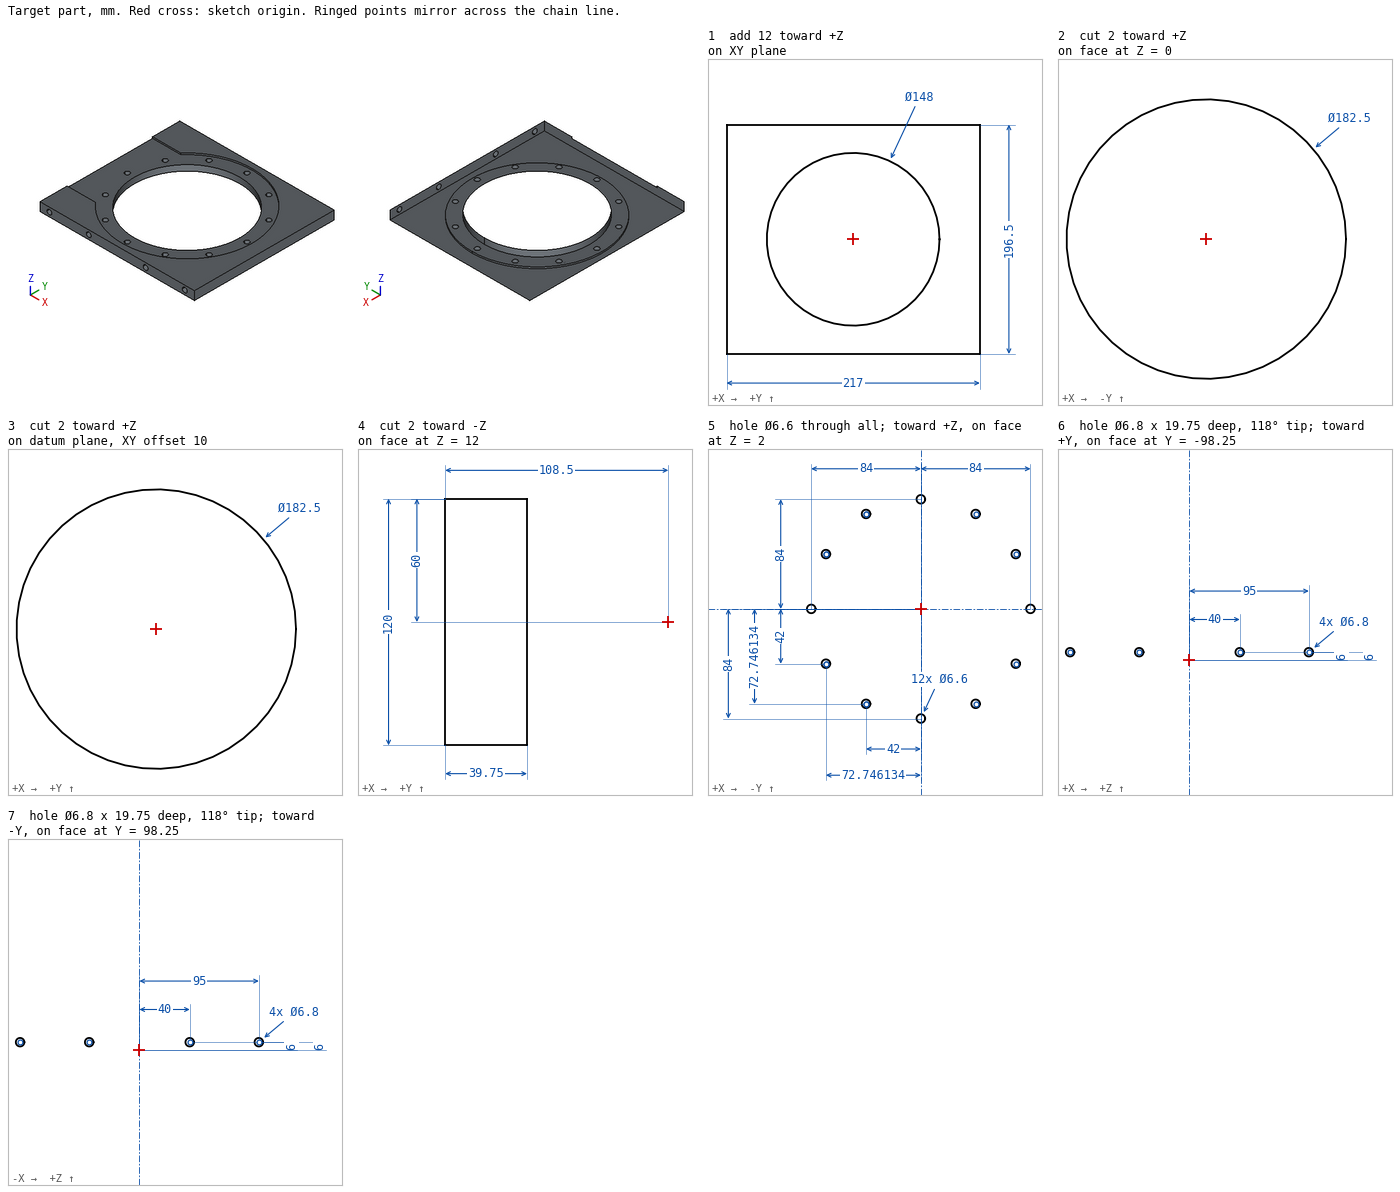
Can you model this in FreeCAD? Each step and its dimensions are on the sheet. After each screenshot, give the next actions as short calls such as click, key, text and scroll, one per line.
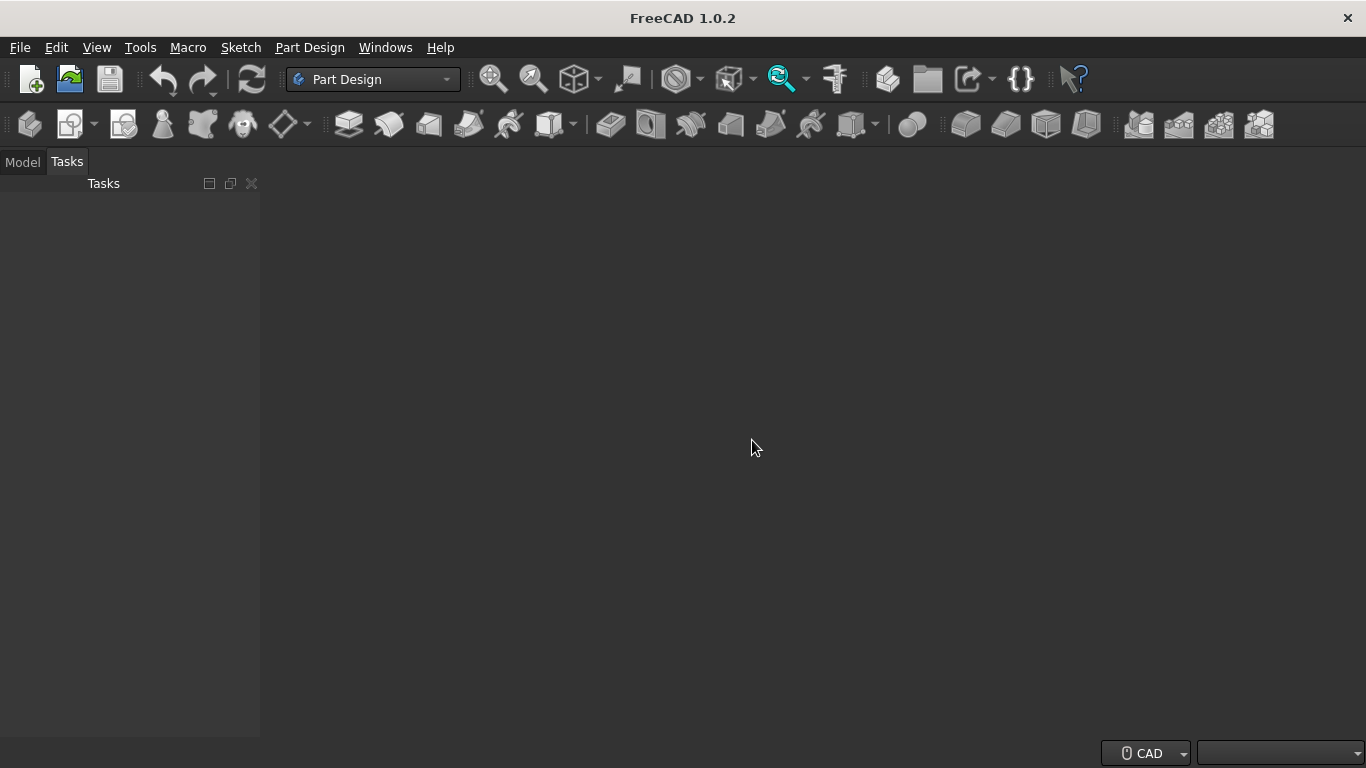
click(30, 80)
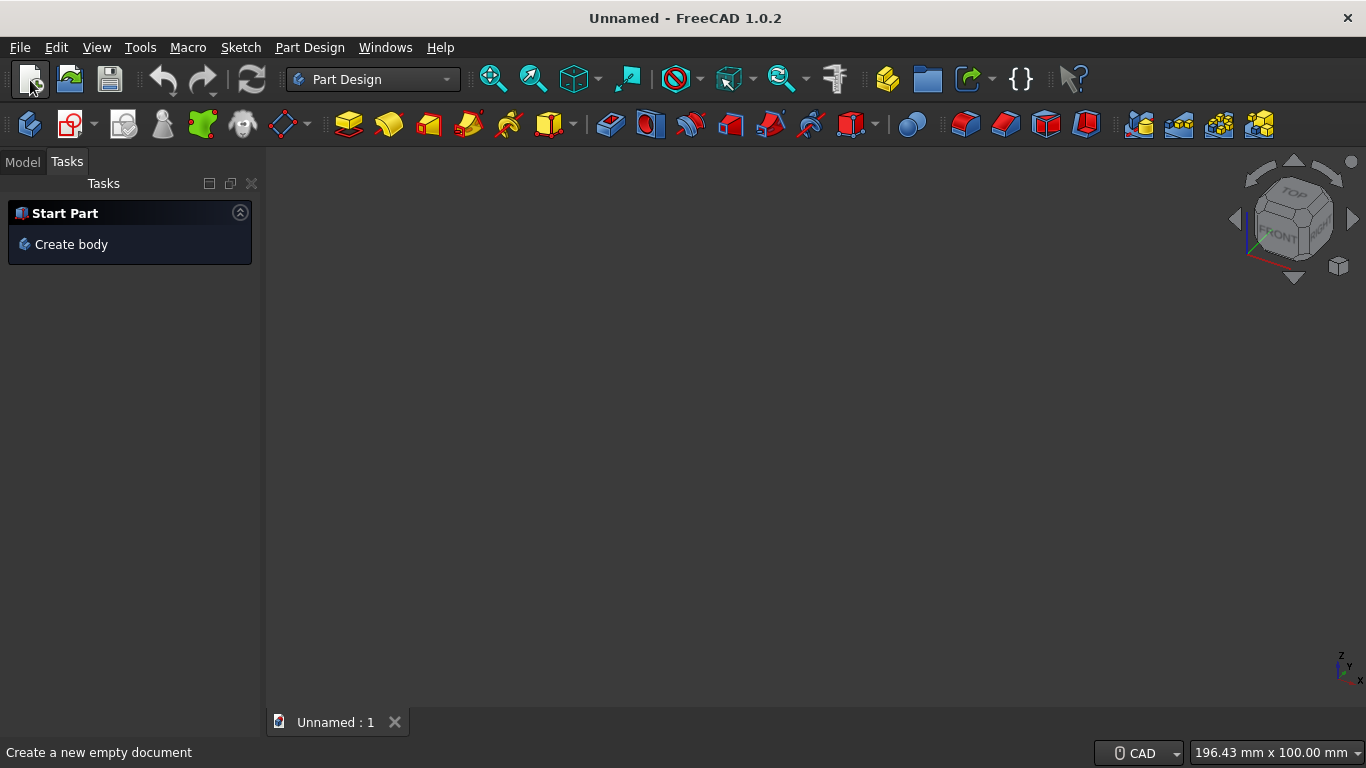
click(70, 124)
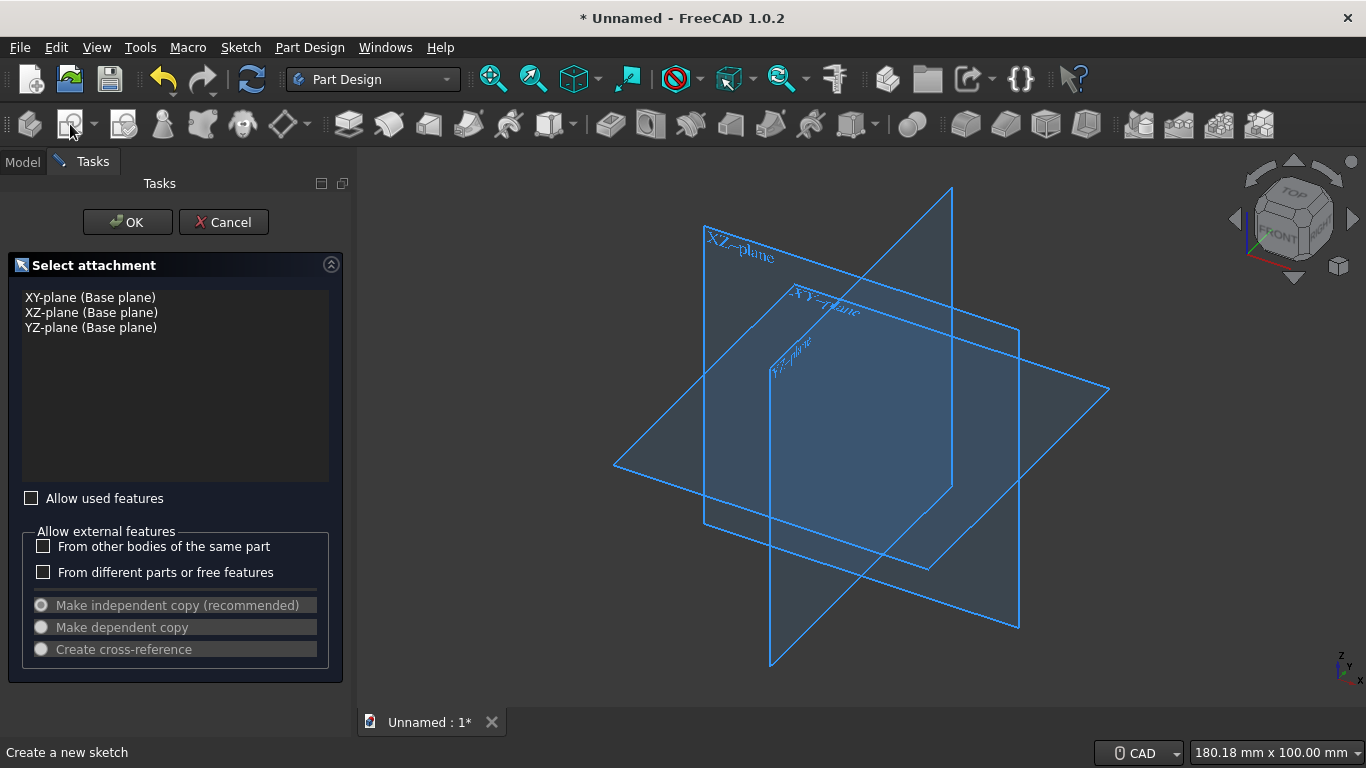
click(82, 298)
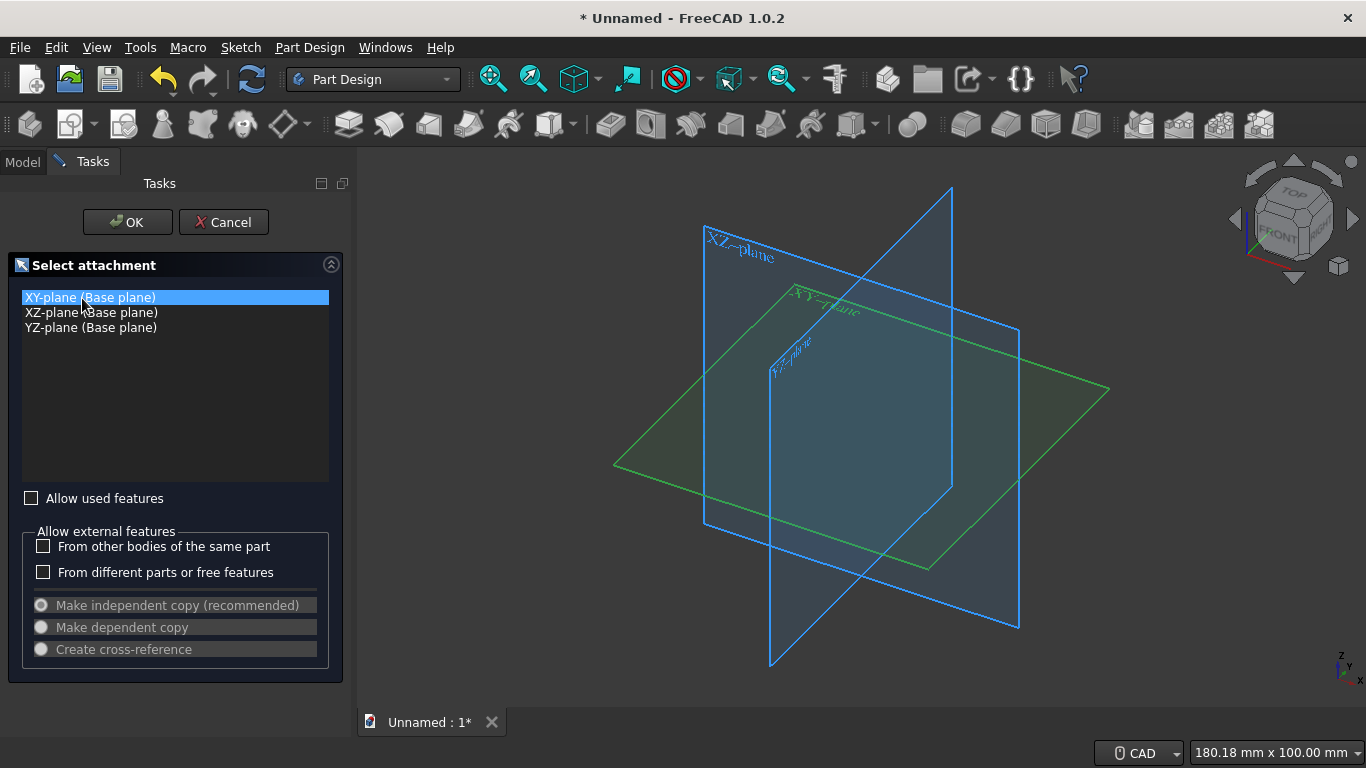
click(128, 222)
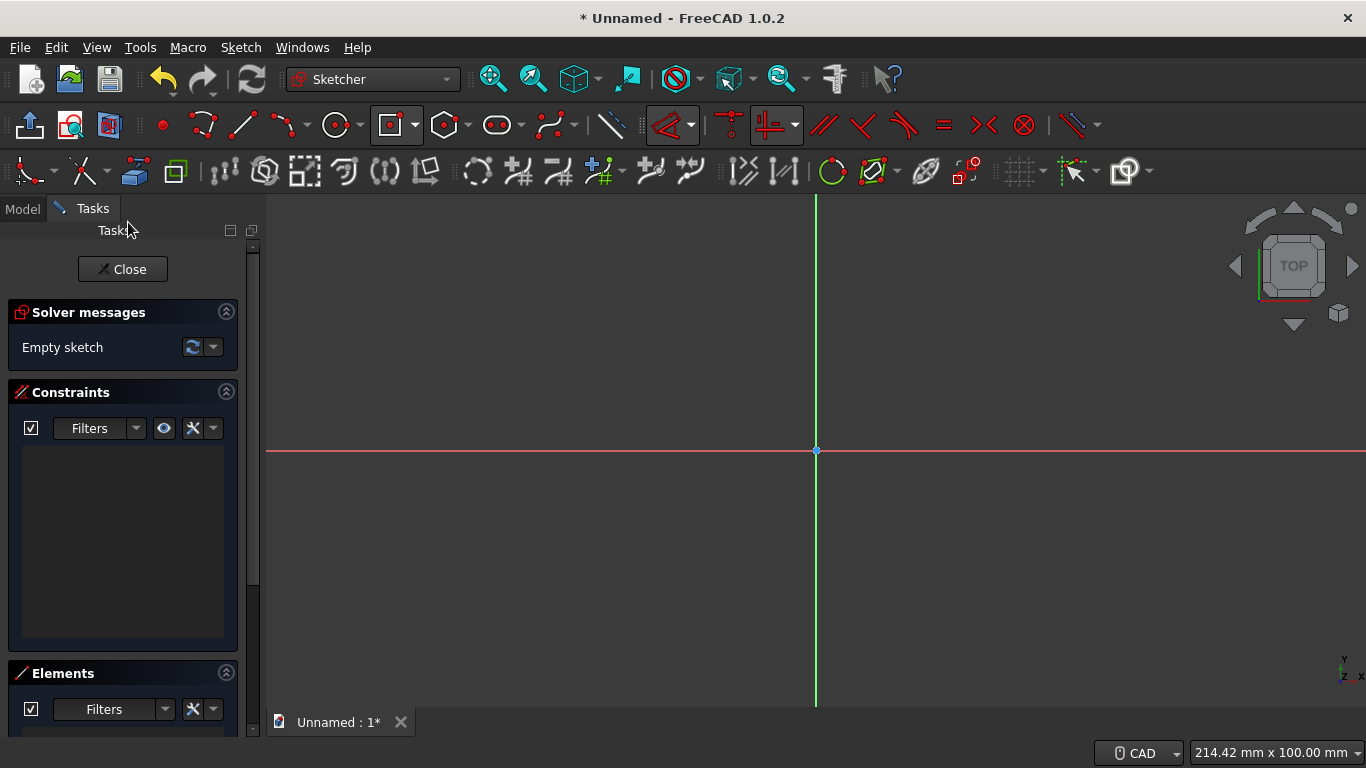
scroll(718, 450, down, 6)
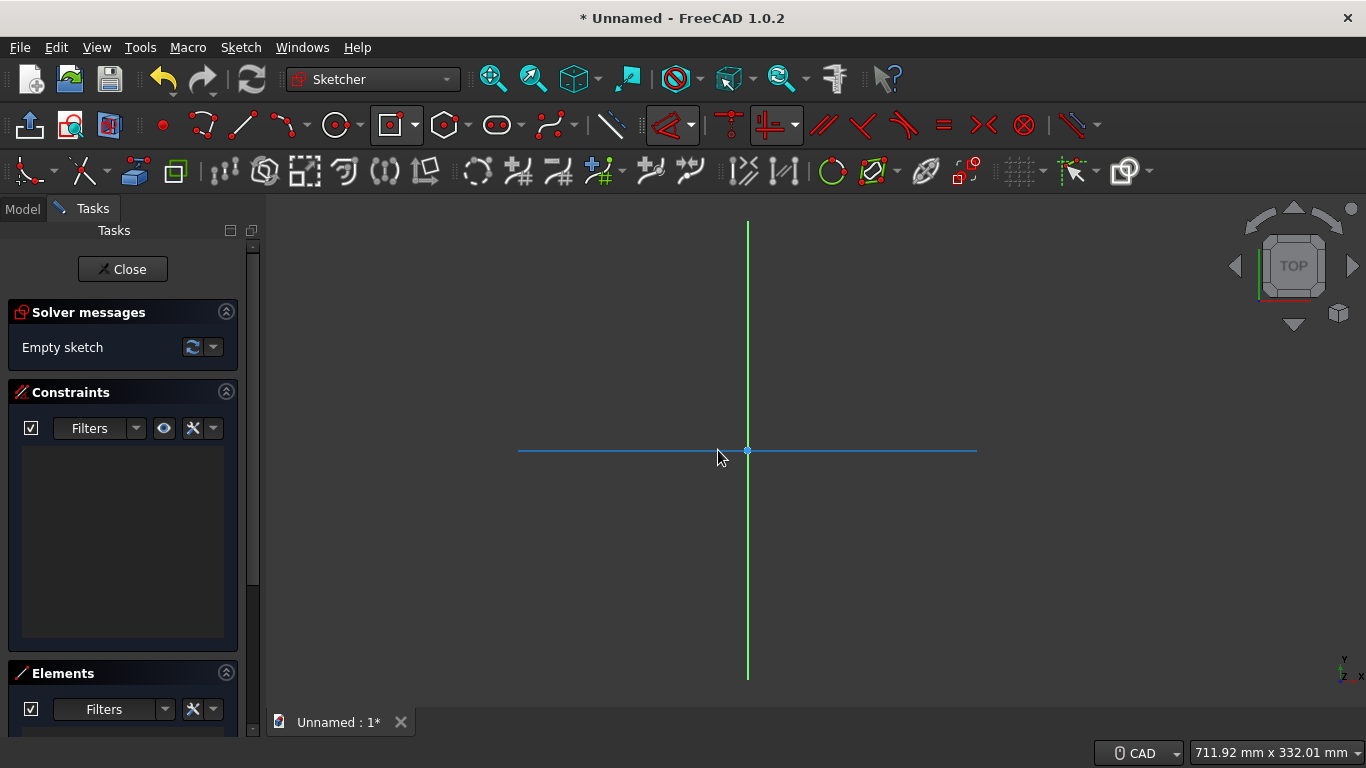
click(390, 126)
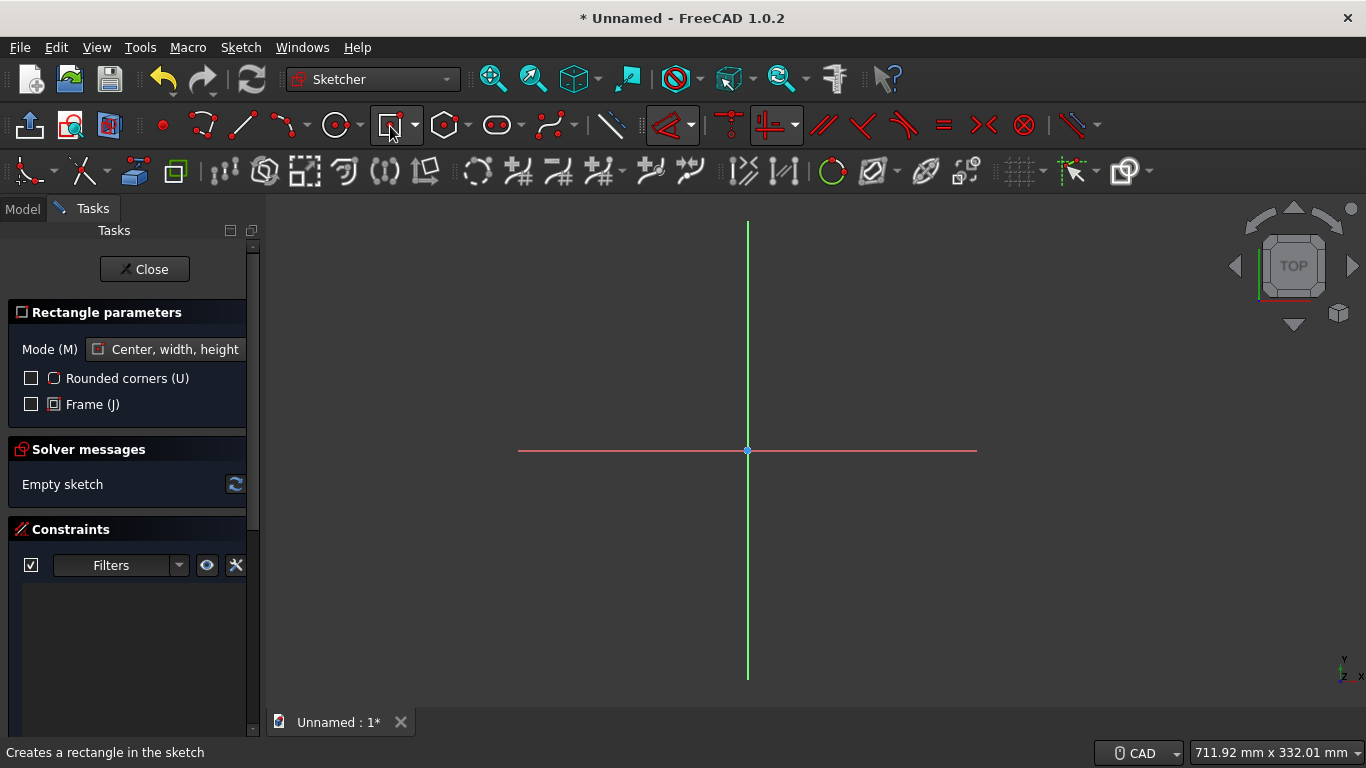
click(748, 450)
click(915, 299)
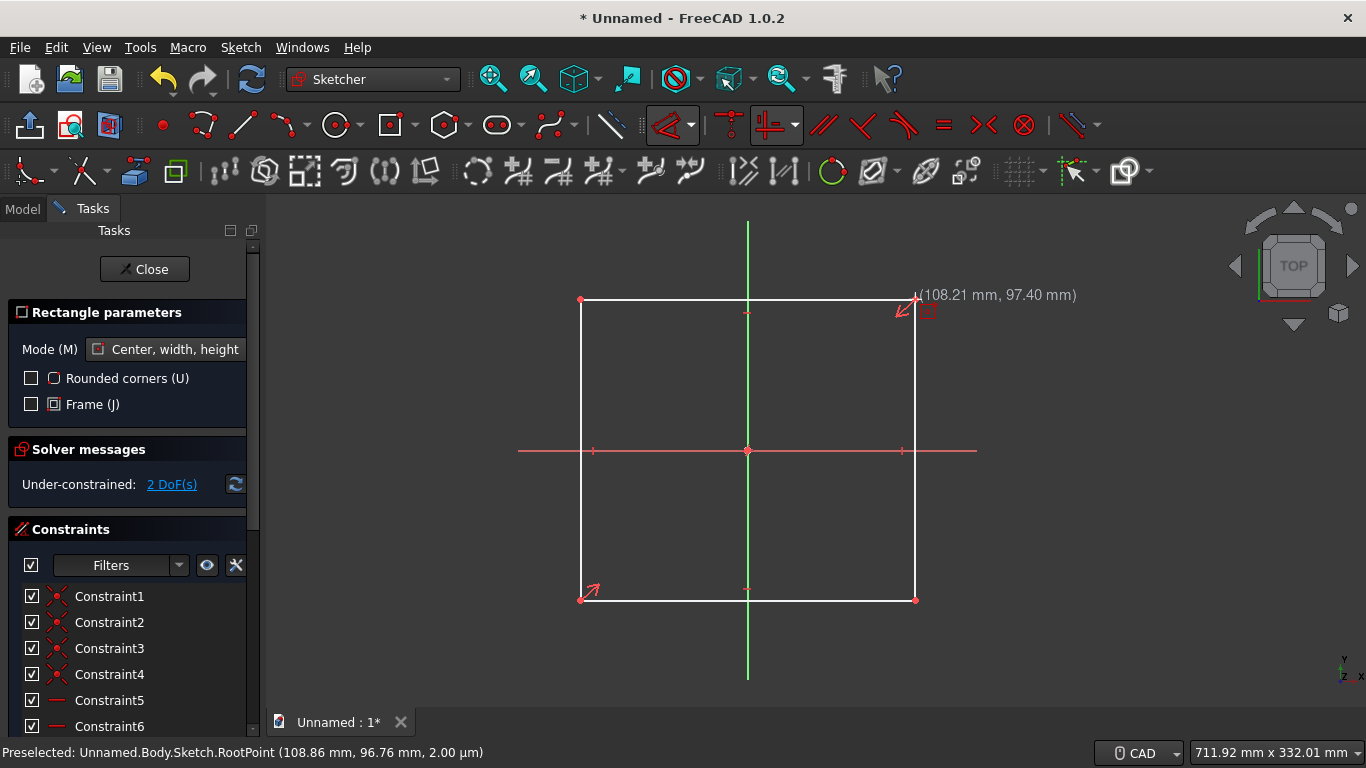
click(336, 126)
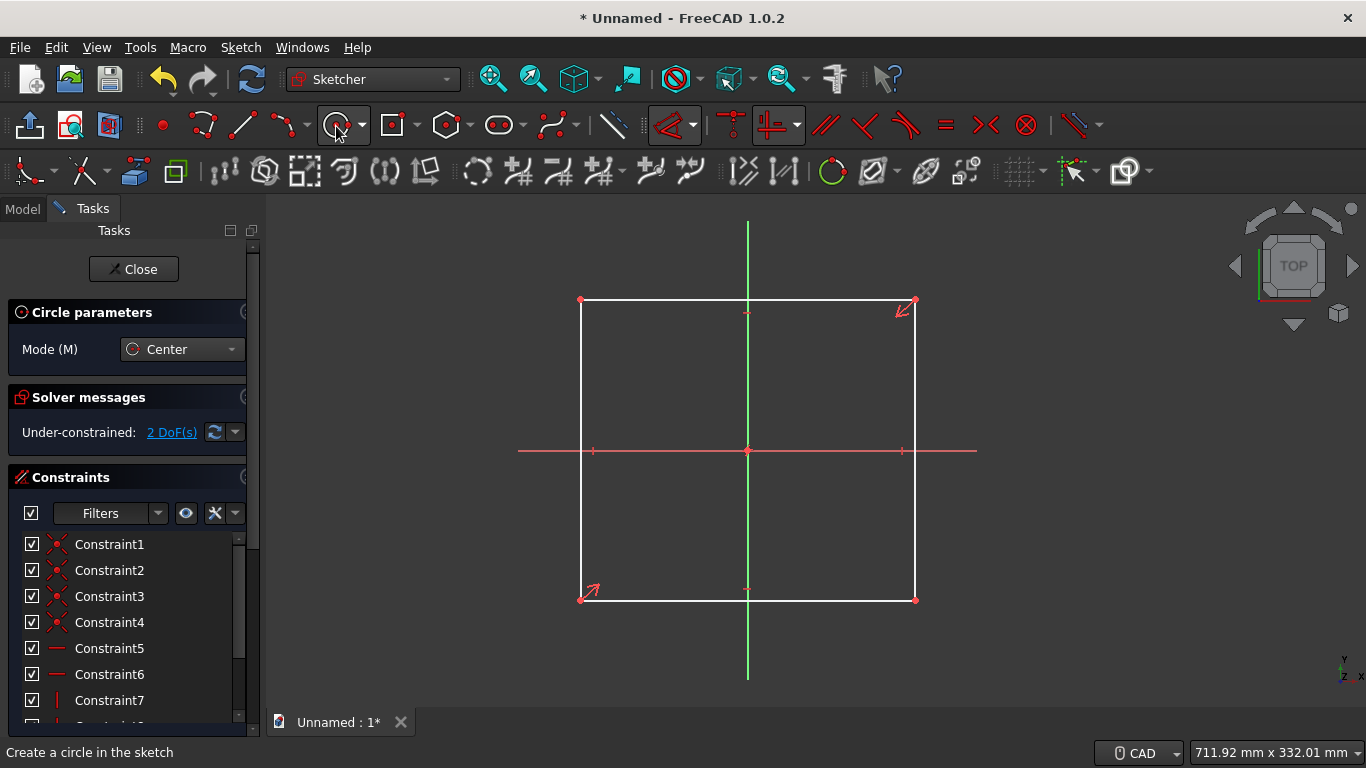
click(748, 450)
click(829, 370)
key(Escape)